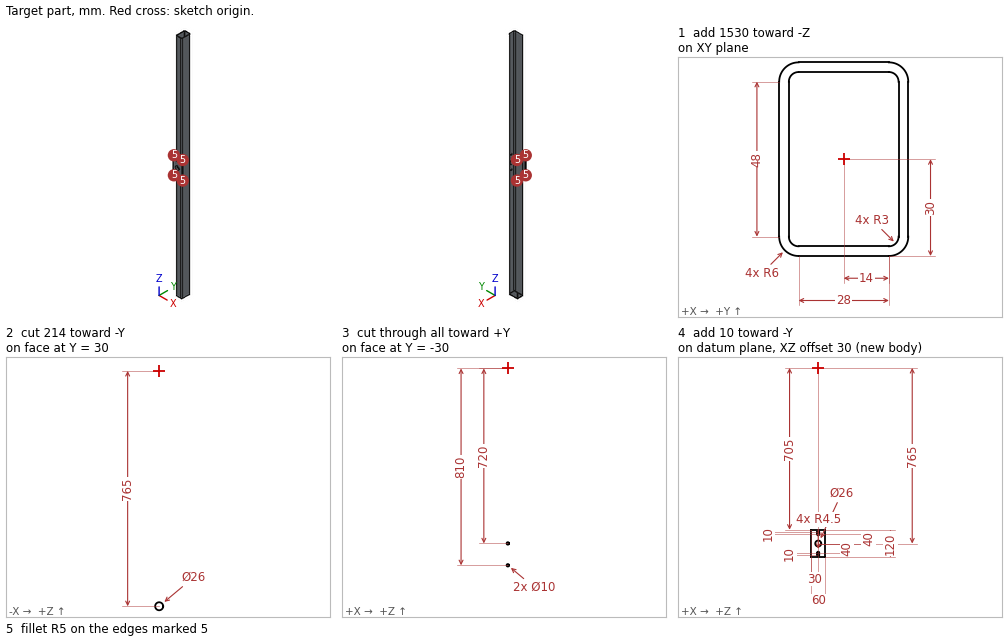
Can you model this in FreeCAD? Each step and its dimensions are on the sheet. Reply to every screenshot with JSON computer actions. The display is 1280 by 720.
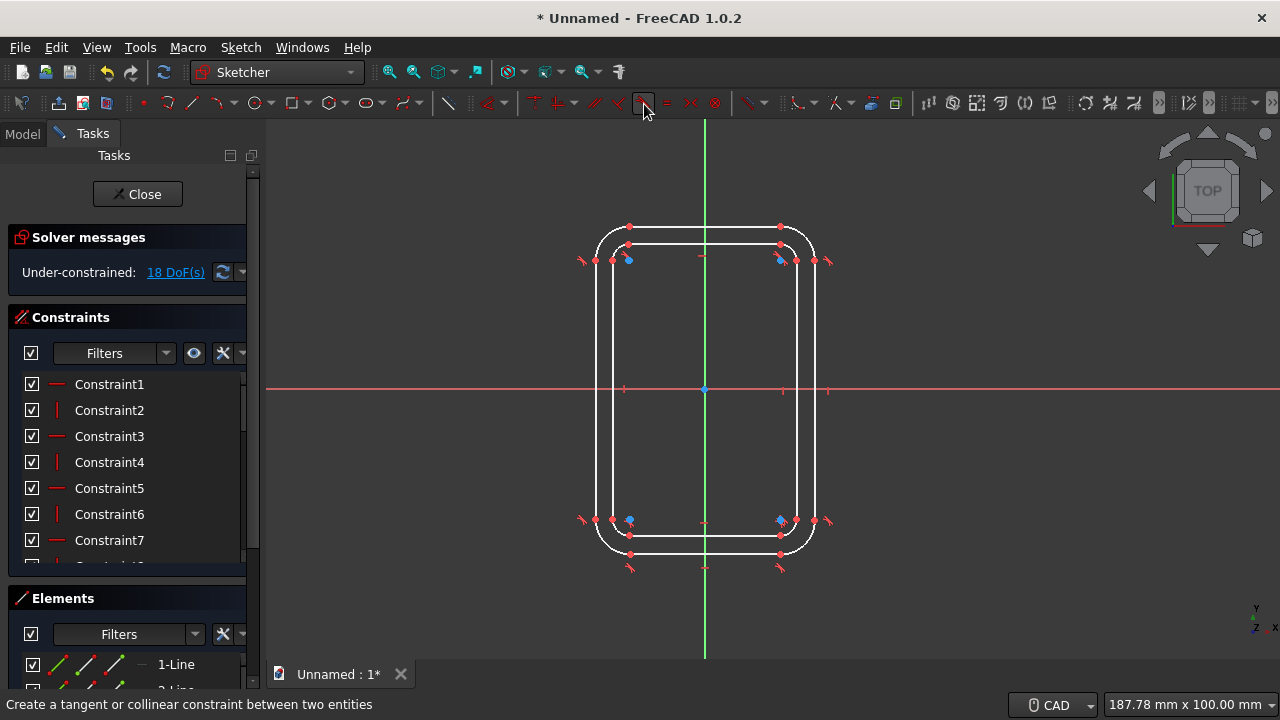
{"action": "left_click", "coordinate": [613, 339]}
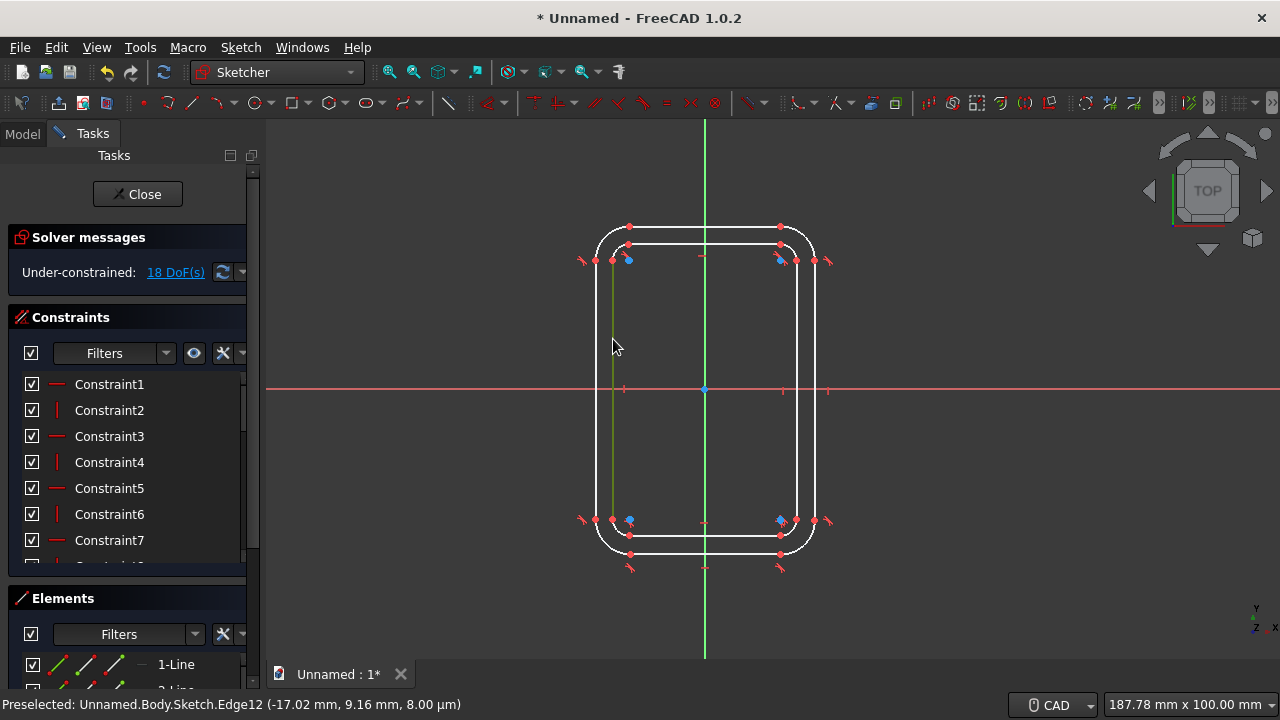
{"action": "left_click", "coordinate": [617, 249]}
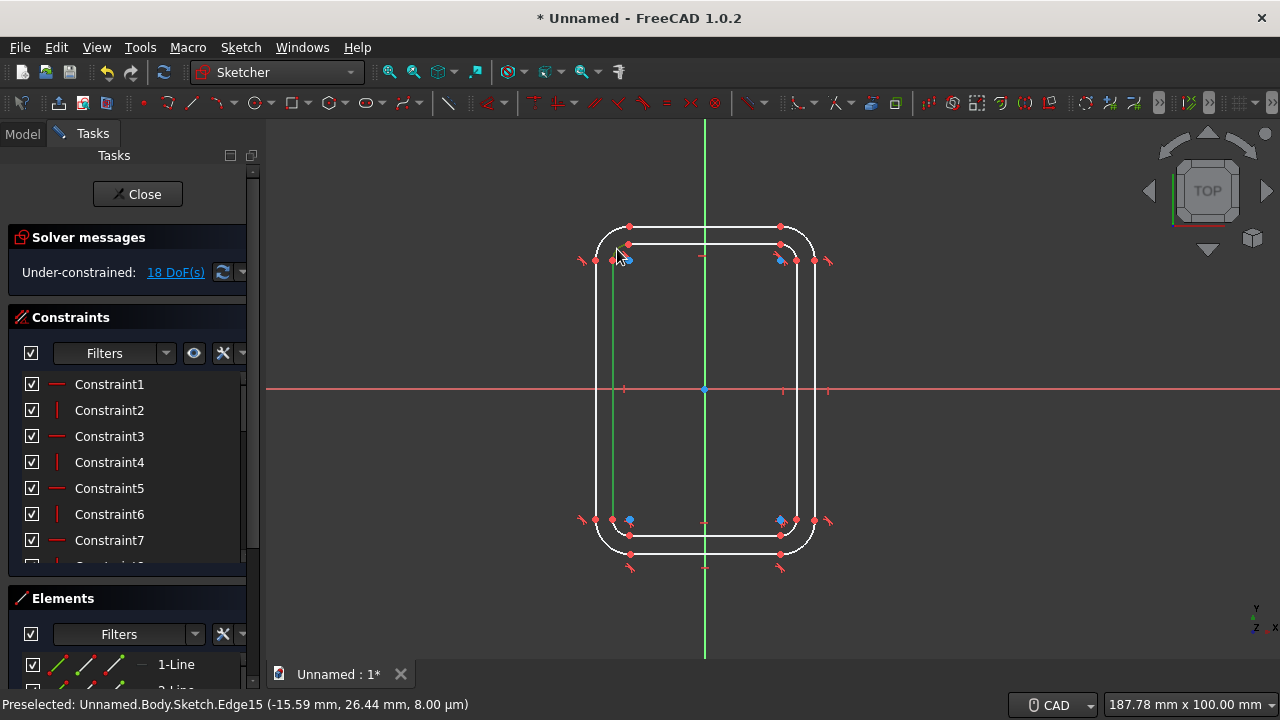
{"action": "left_click", "coordinate": [644, 104]}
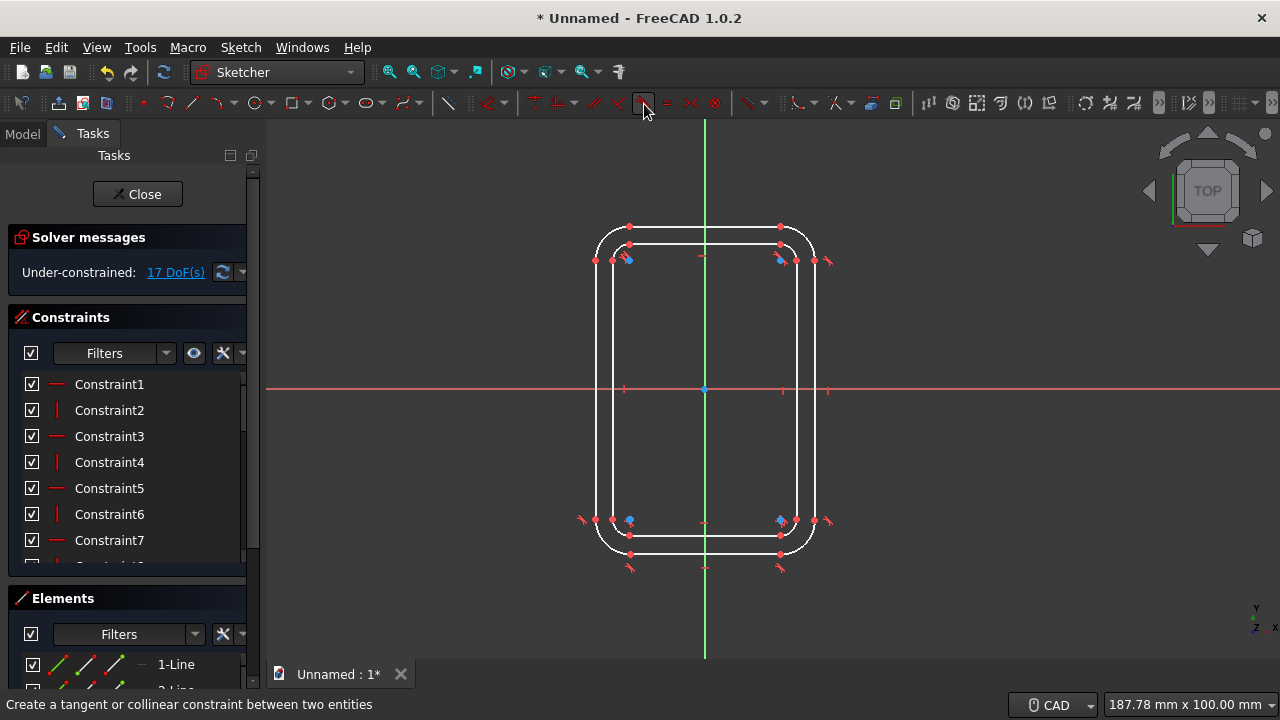
{"action": "left_click", "coordinate": [613, 339]}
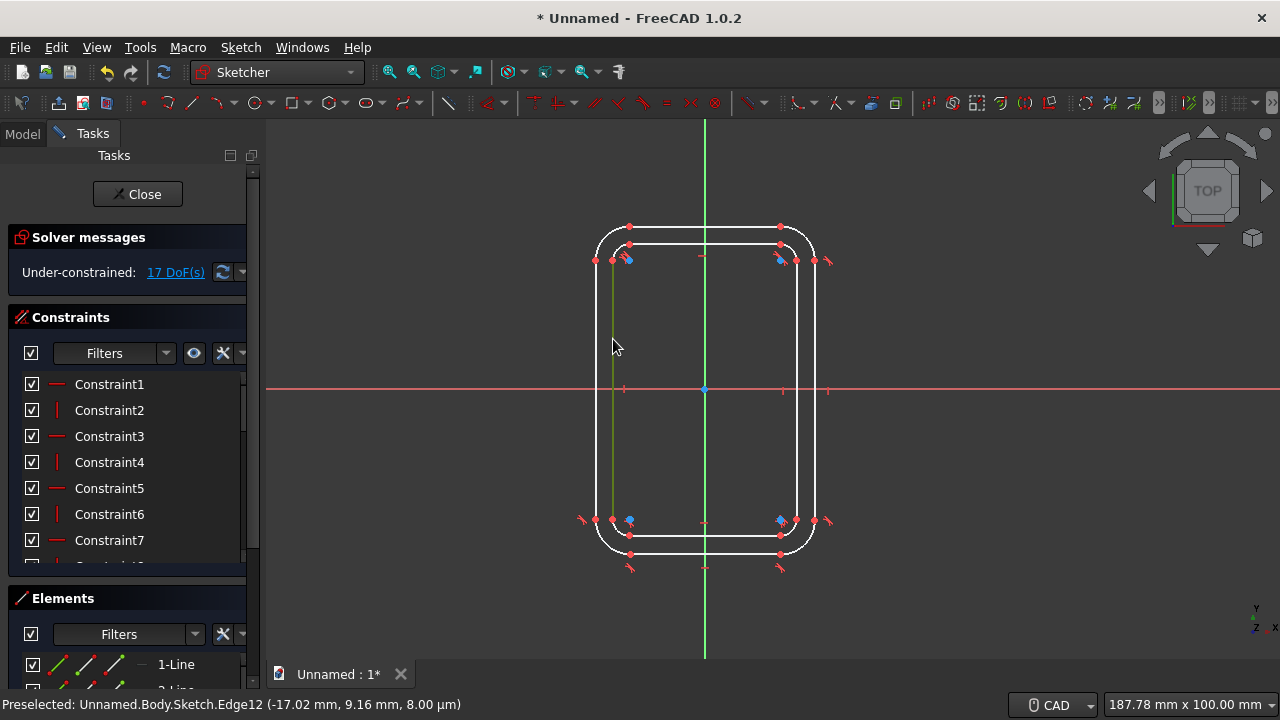
{"action": "left_click", "coordinate": [618, 531]}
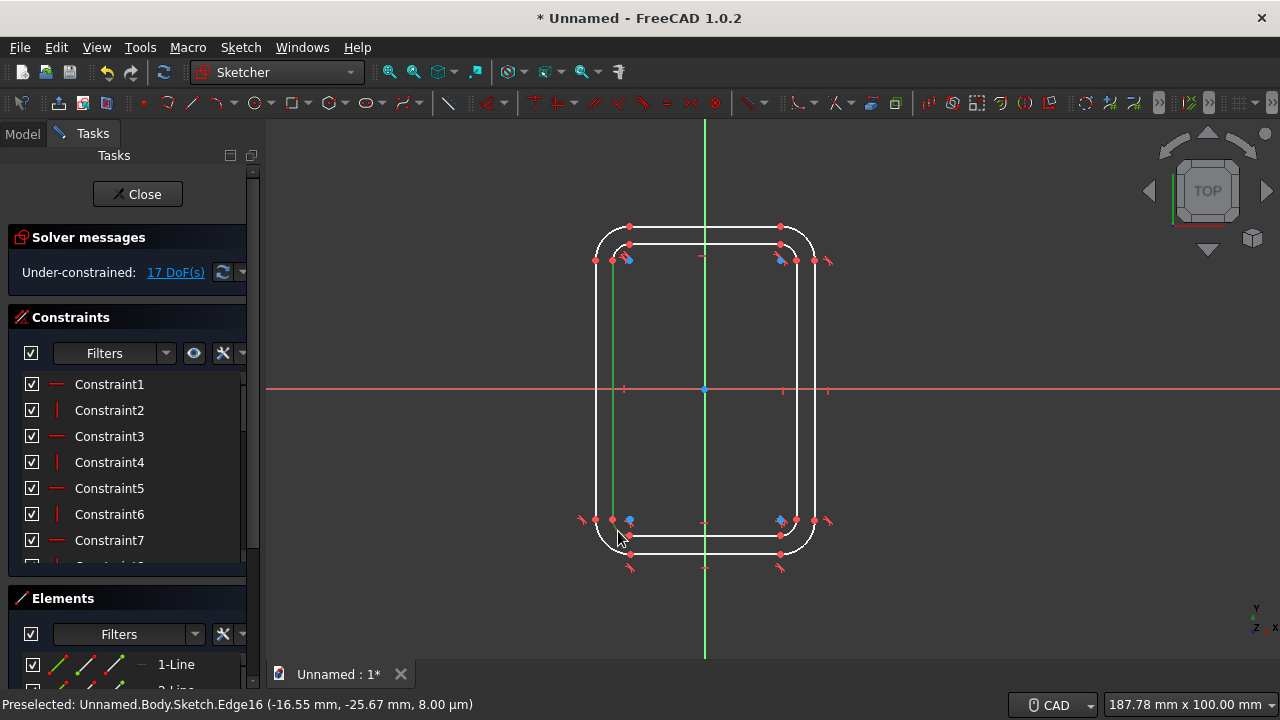
{"action": "left_click", "coordinate": [644, 104]}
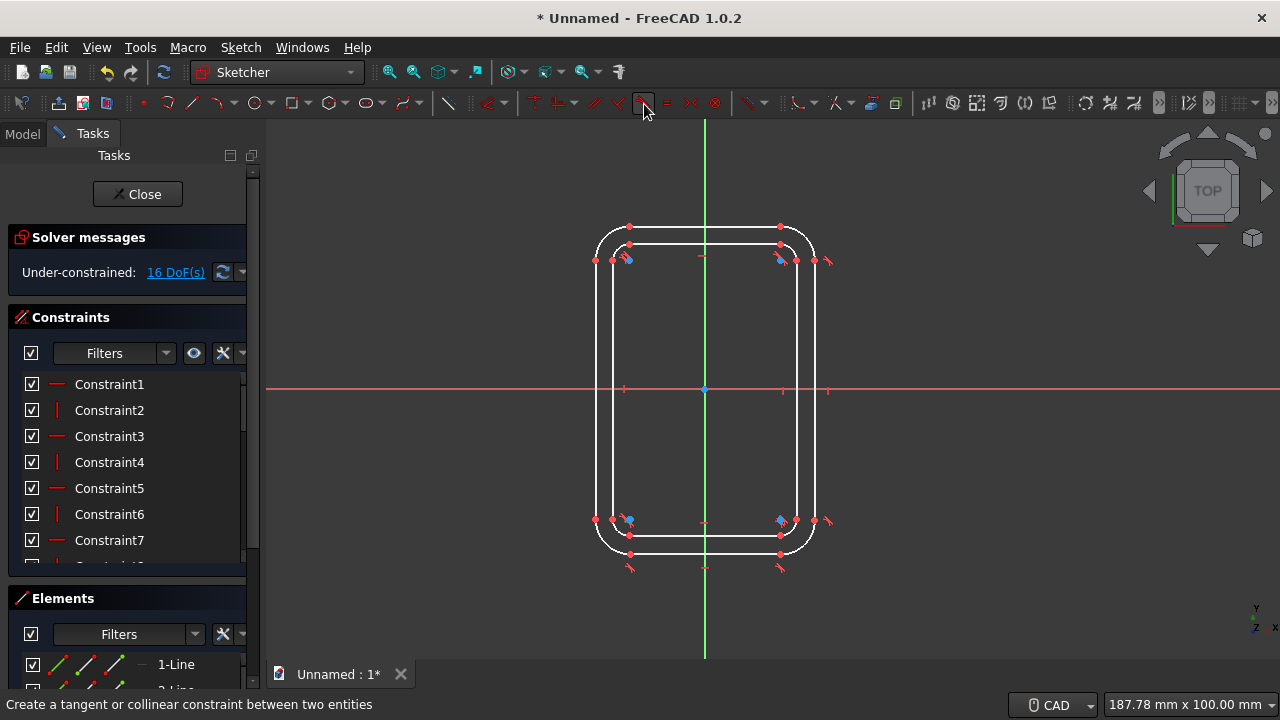
{"action": "left_click", "coordinate": [796, 551]}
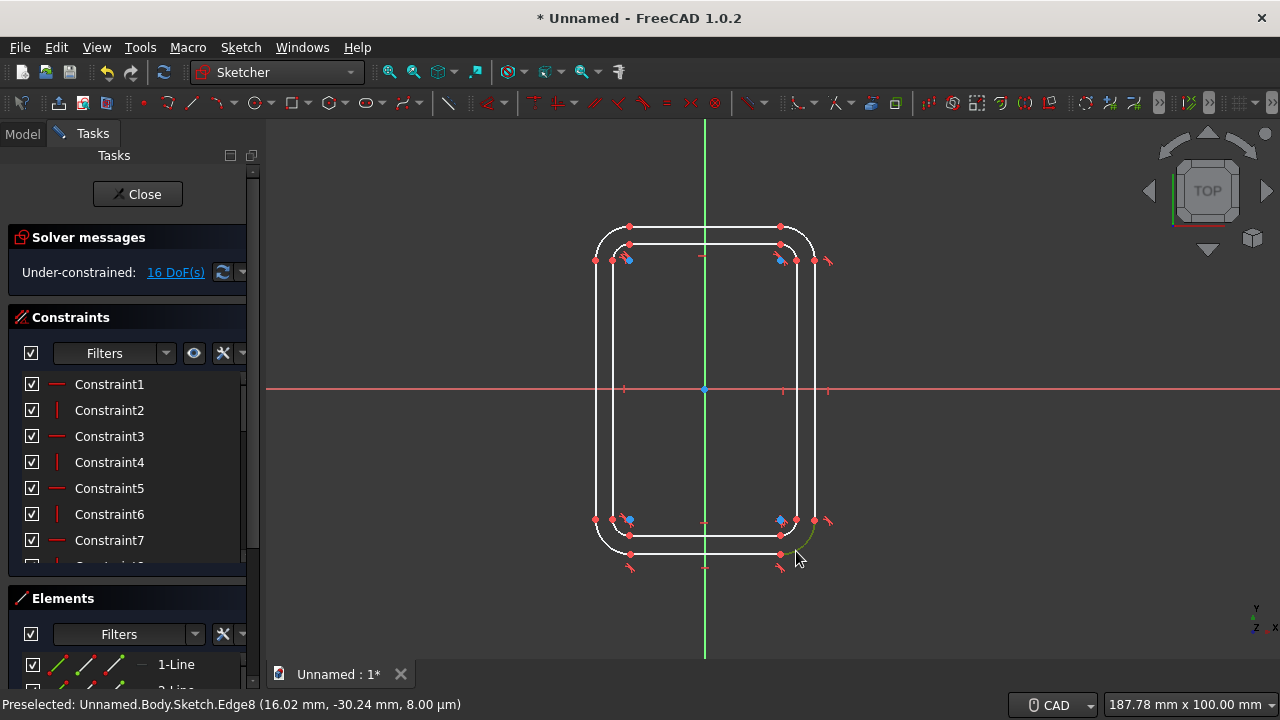
{"action": "left_click", "coordinate": [792, 531]}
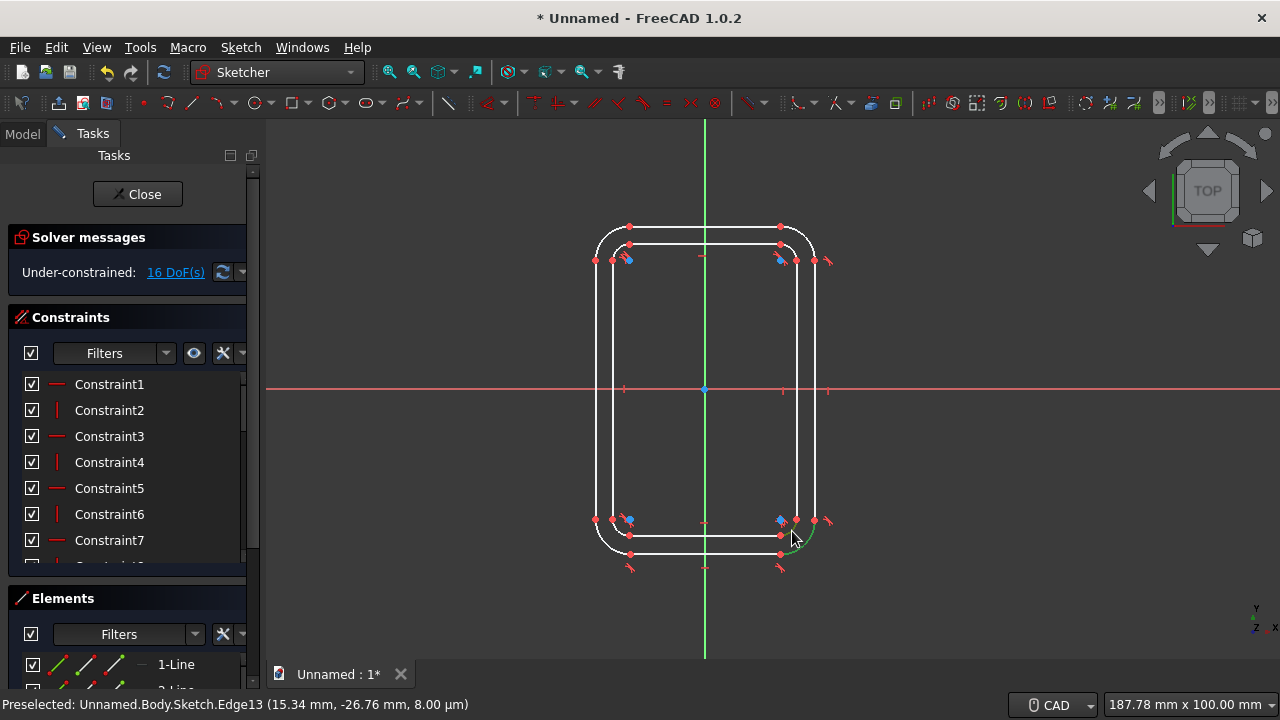
{"action": "left_click", "coordinate": [534, 104]}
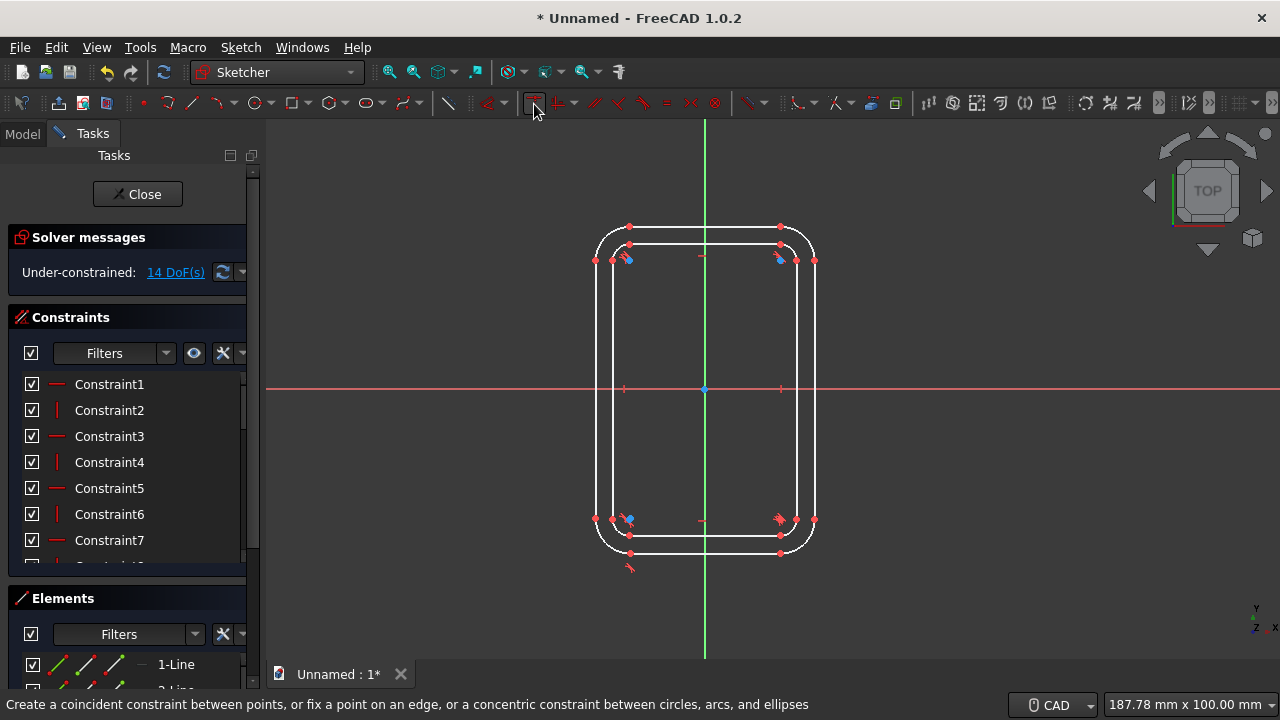
{"action": "left_click", "coordinate": [811, 245]}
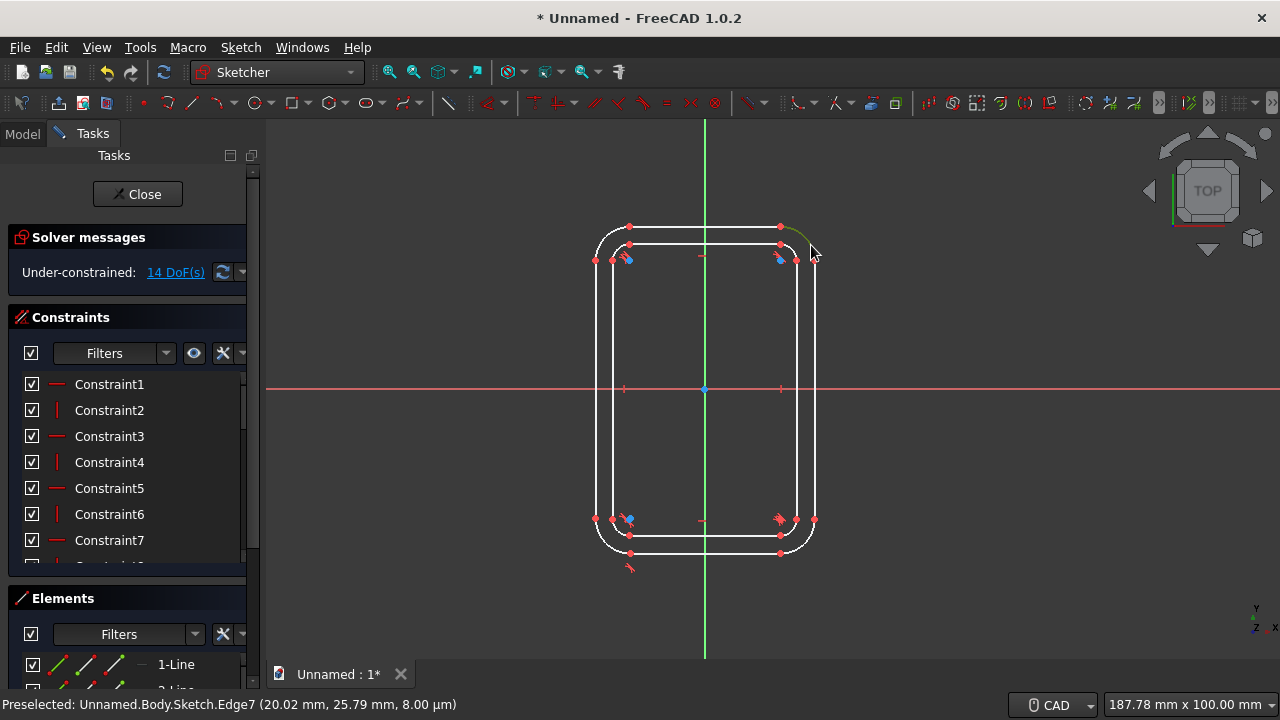
{"action": "left_click", "coordinate": [792, 249]}